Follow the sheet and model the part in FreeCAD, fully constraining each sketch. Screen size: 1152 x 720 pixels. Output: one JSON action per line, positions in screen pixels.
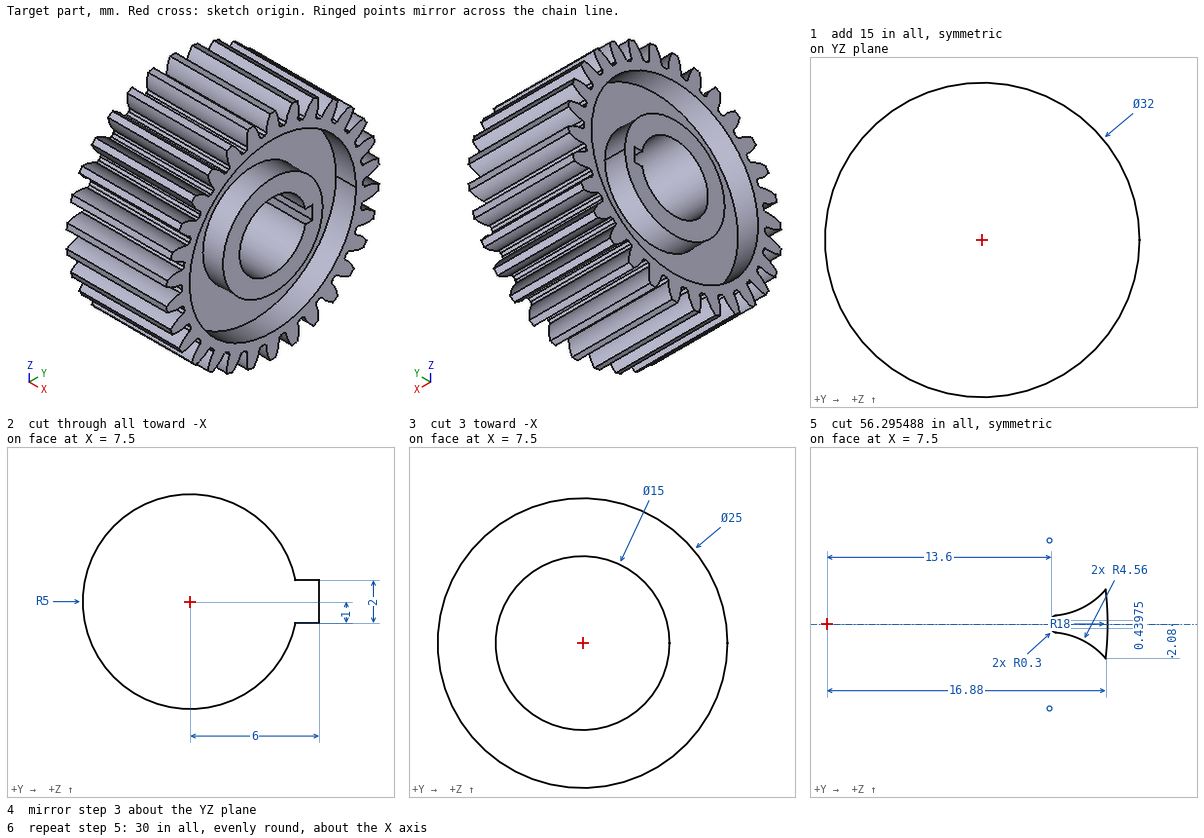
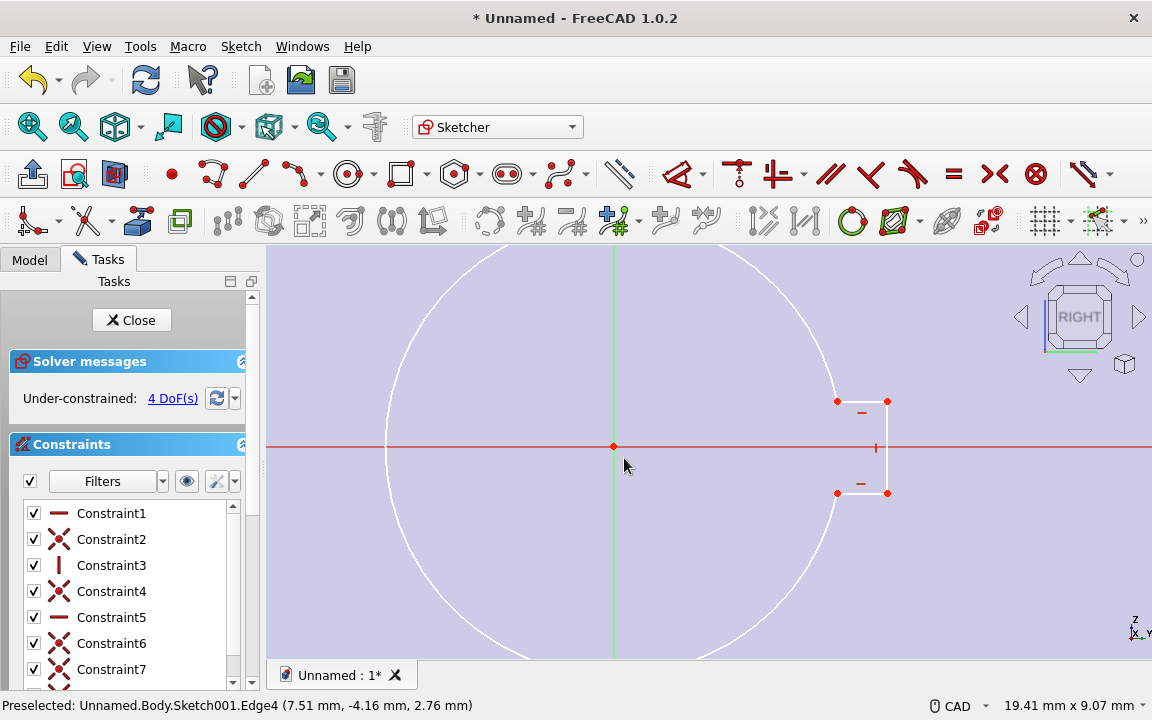
{"action": "left_click", "coordinate": [385, 446]}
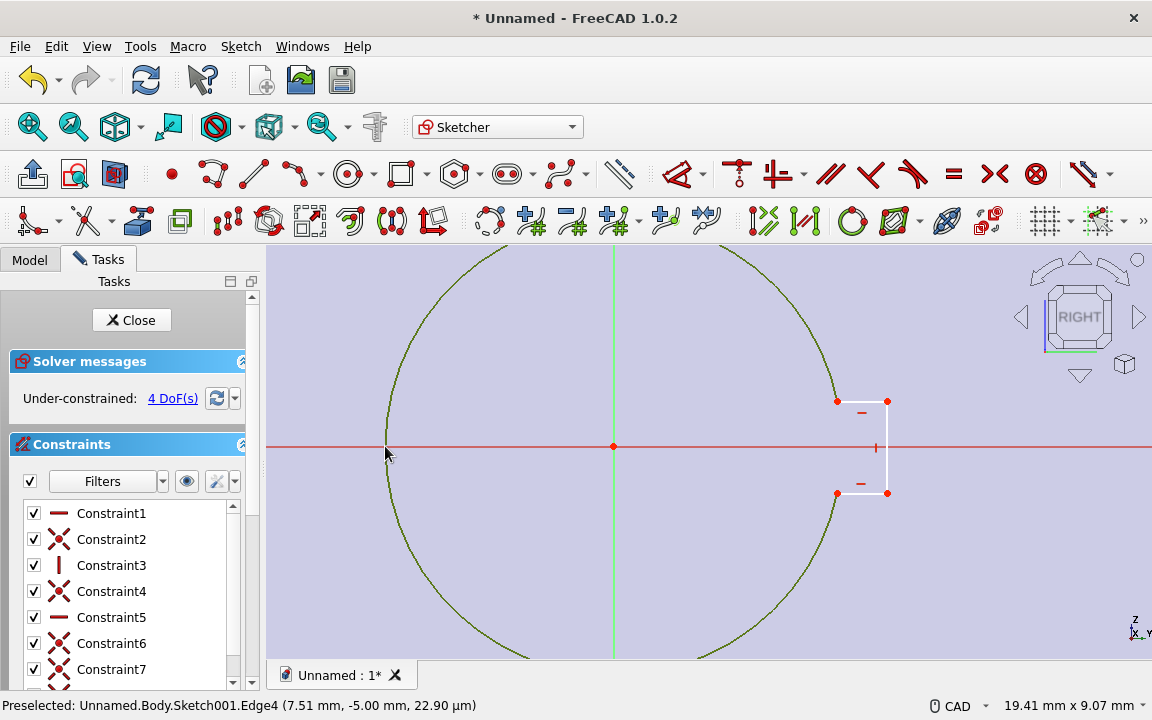
{"action": "key", "text": "k r"}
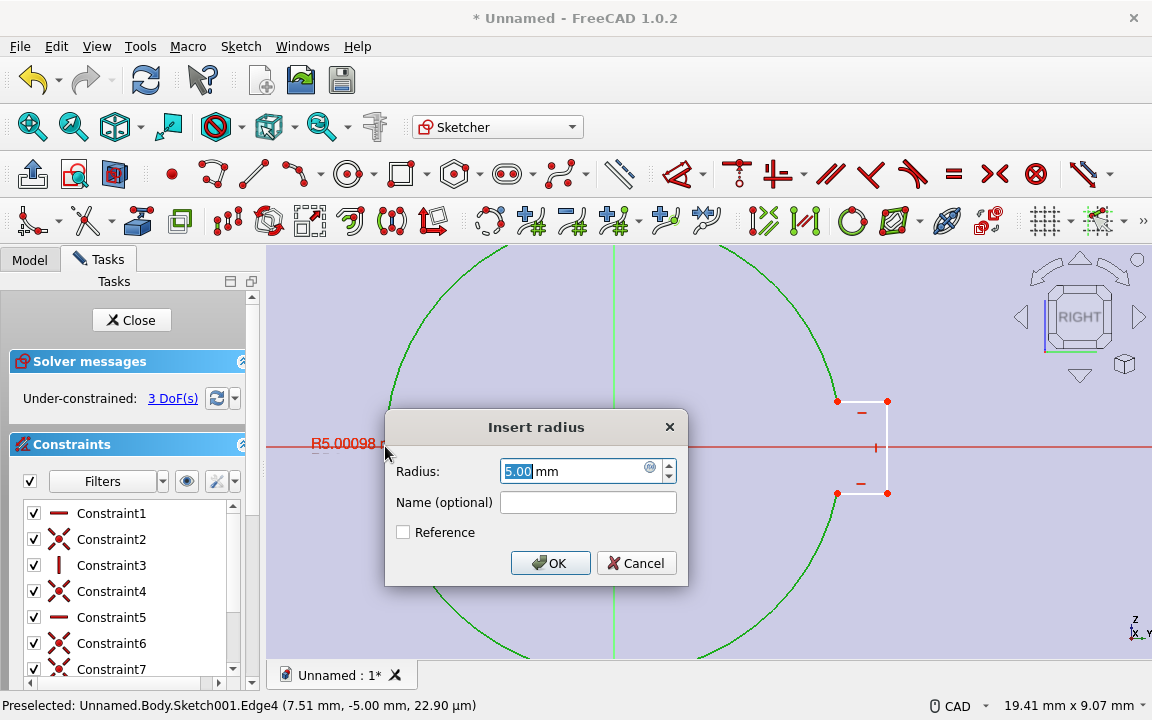
{"action": "type", "text": "5"}
{"action": "key", "text": "Return"}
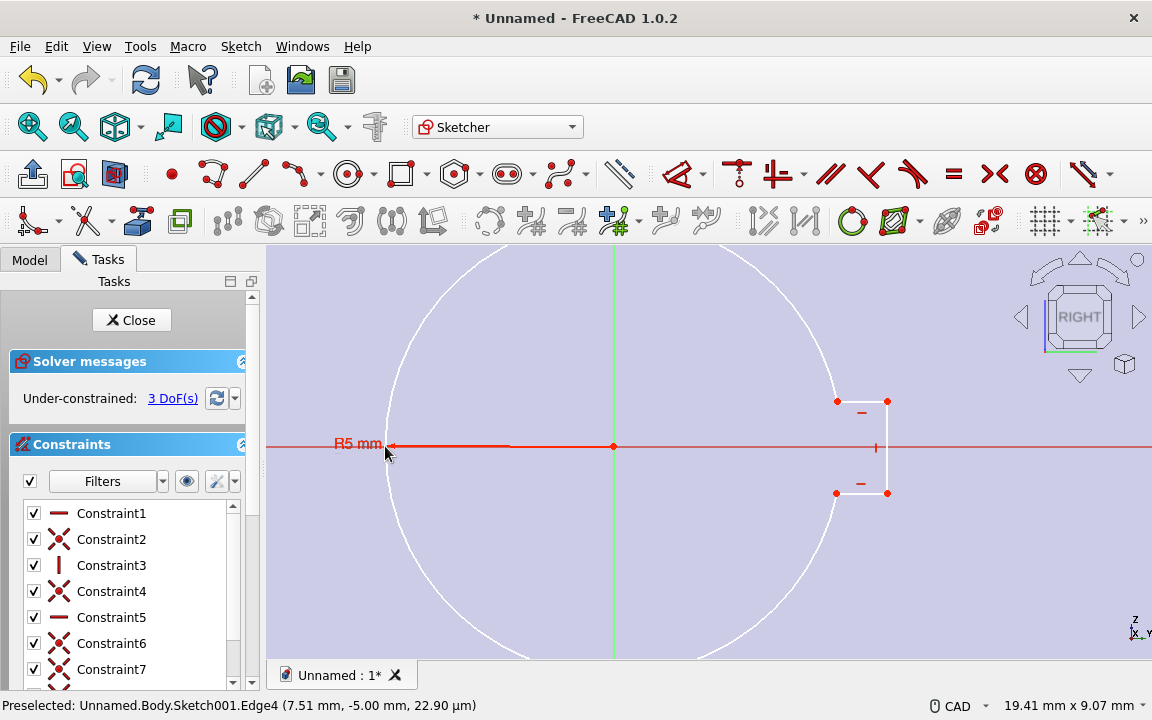
{"action": "left_click", "coordinate": [887, 466]}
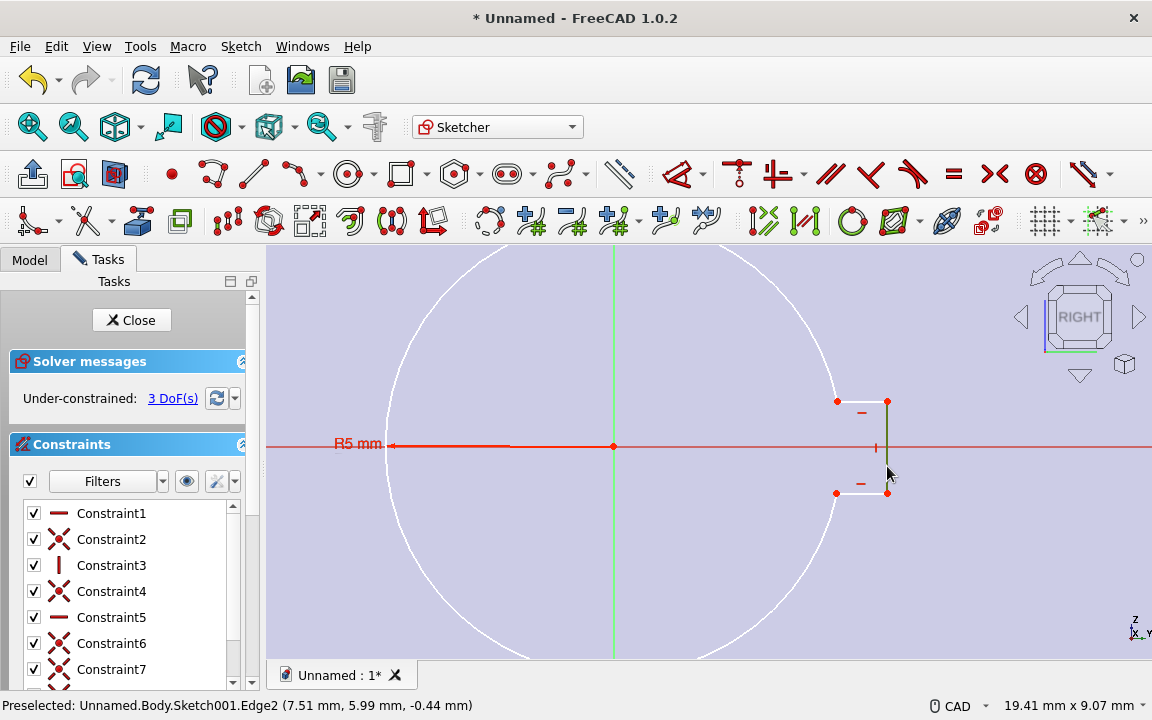
{"action": "key", "text": "i"}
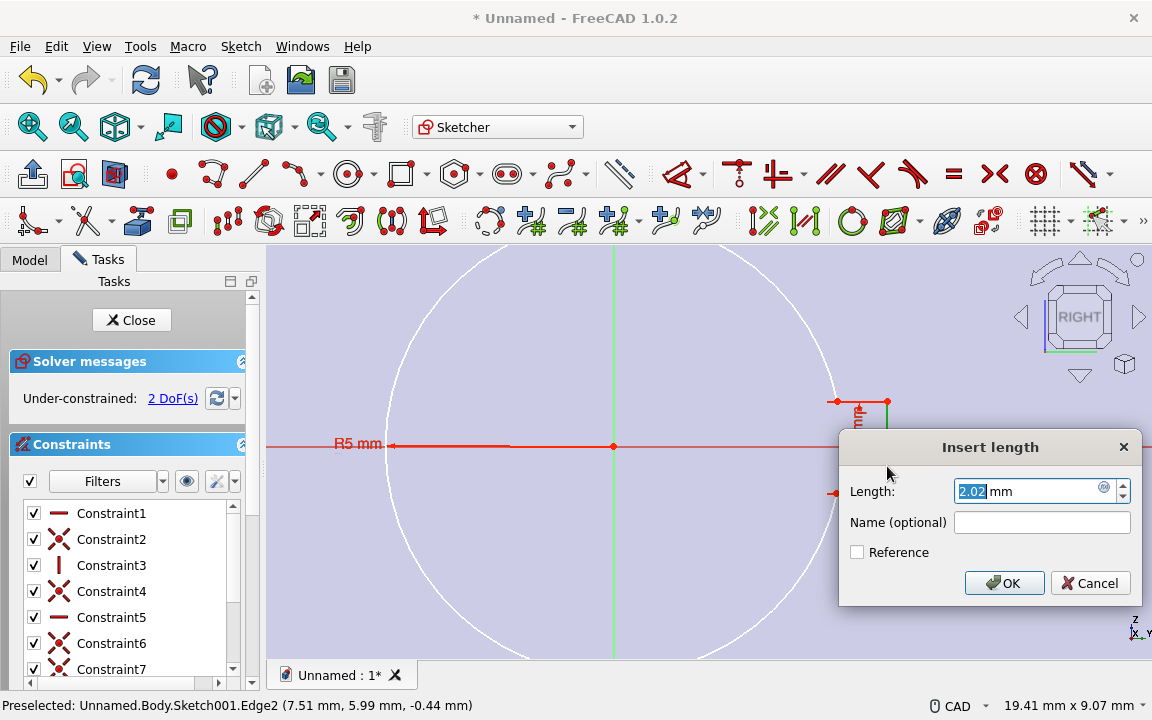
{"action": "type", "text": "2"}
{"action": "key", "text": "Return"}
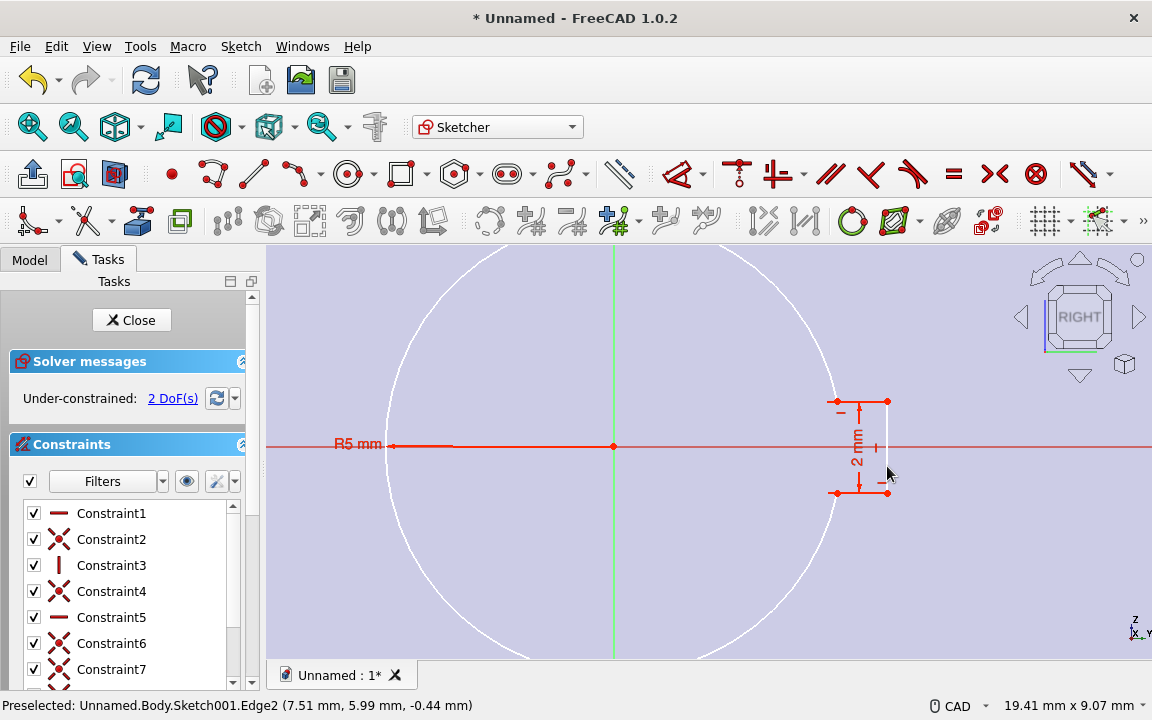
{"action": "left_click", "coordinate": [837, 493]}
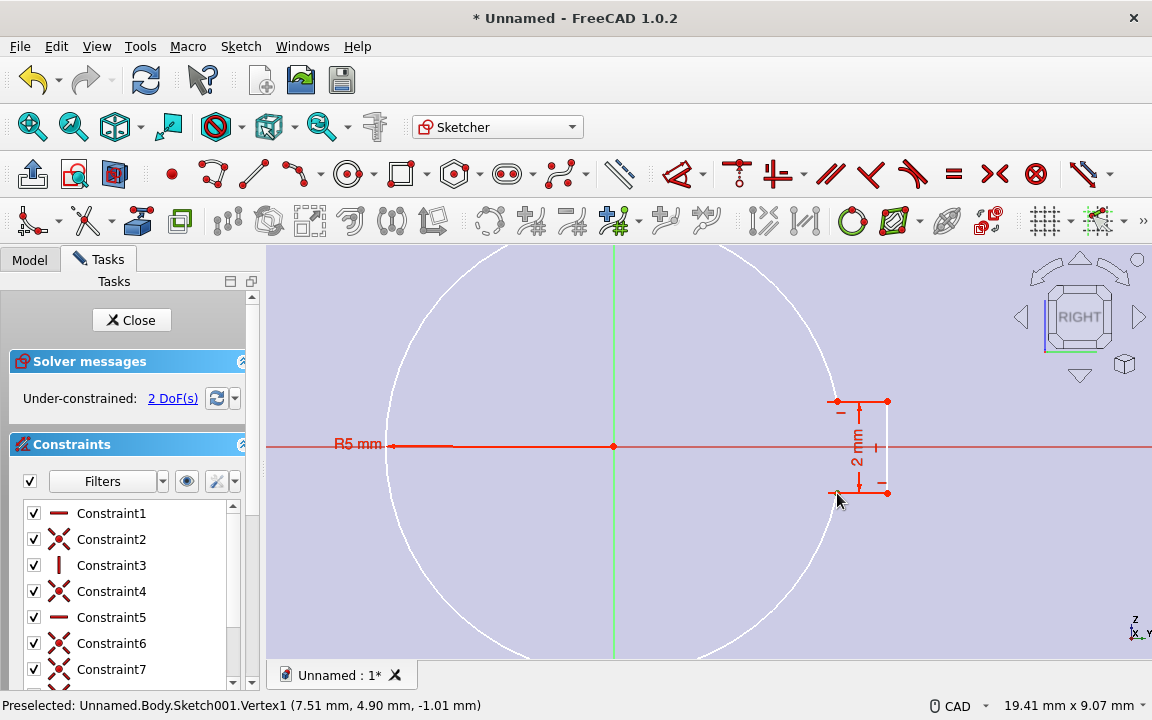
{"action": "key", "text": "i"}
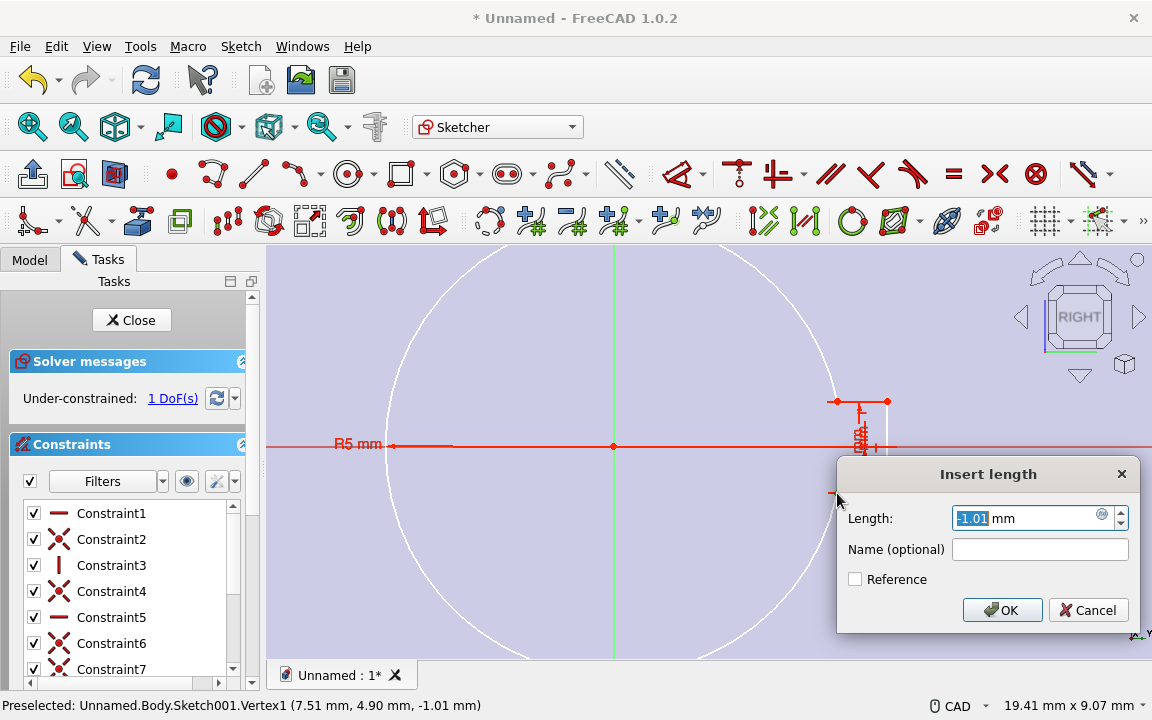
{"action": "type", "text": "-1"}
{"action": "key", "text": "Return"}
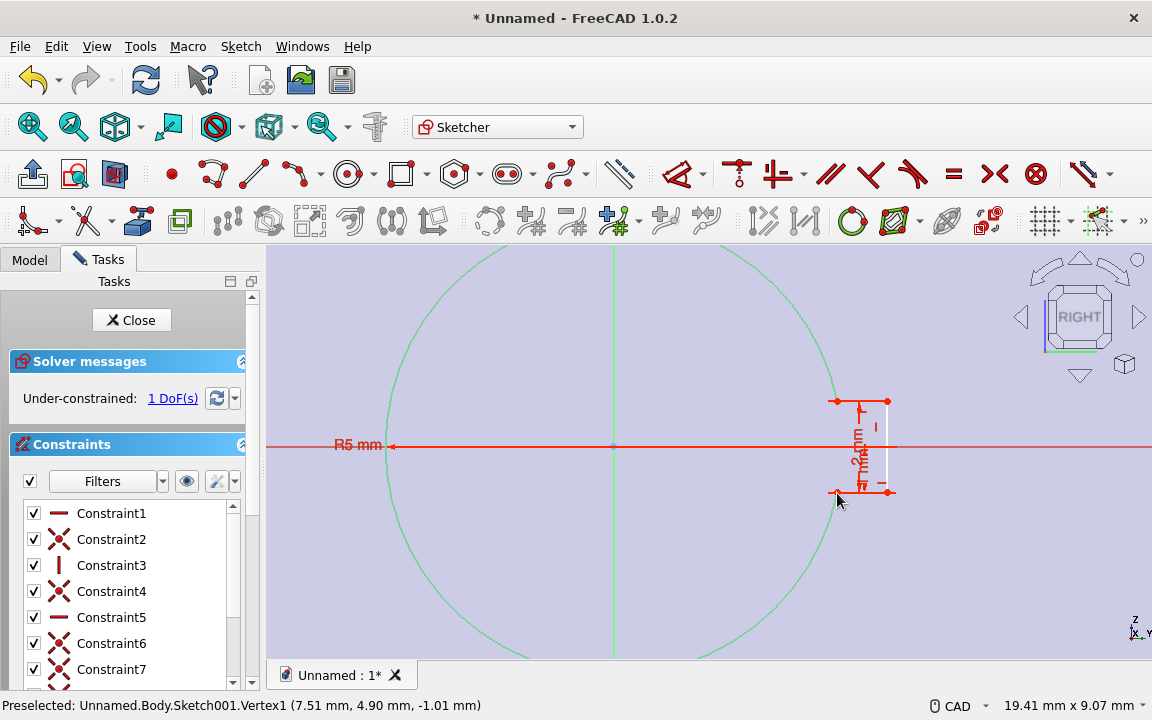
{"action": "left_click", "coordinate": [887, 493]}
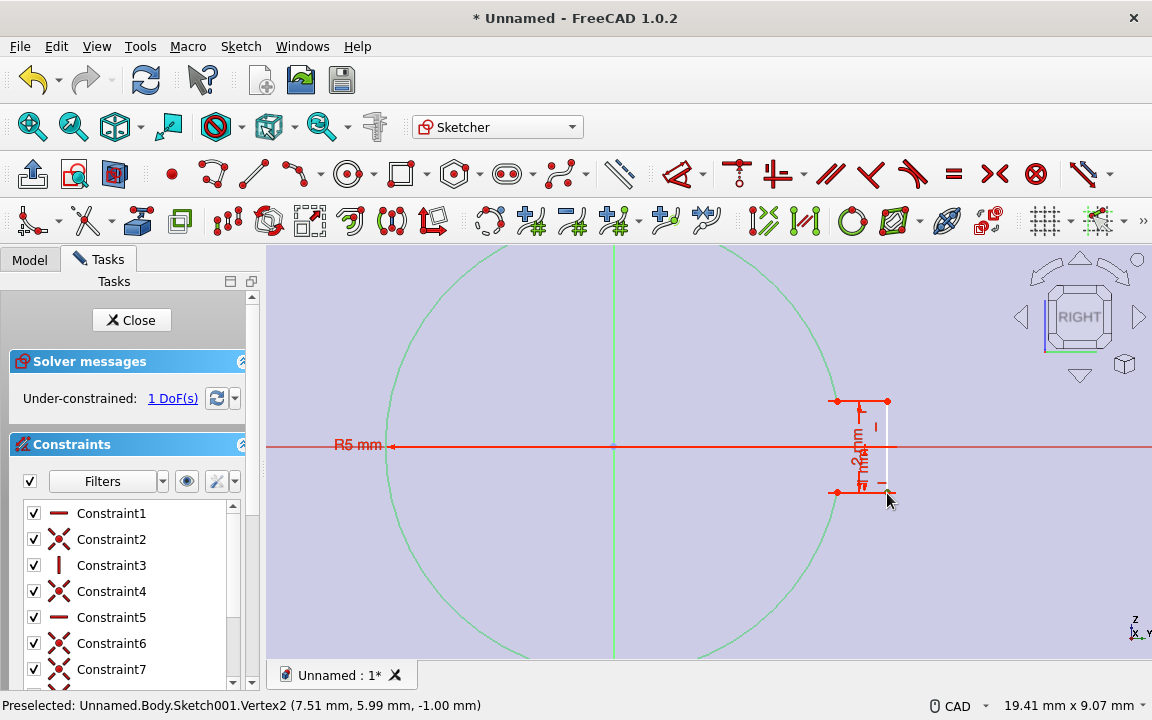
{"action": "key", "text": "l"}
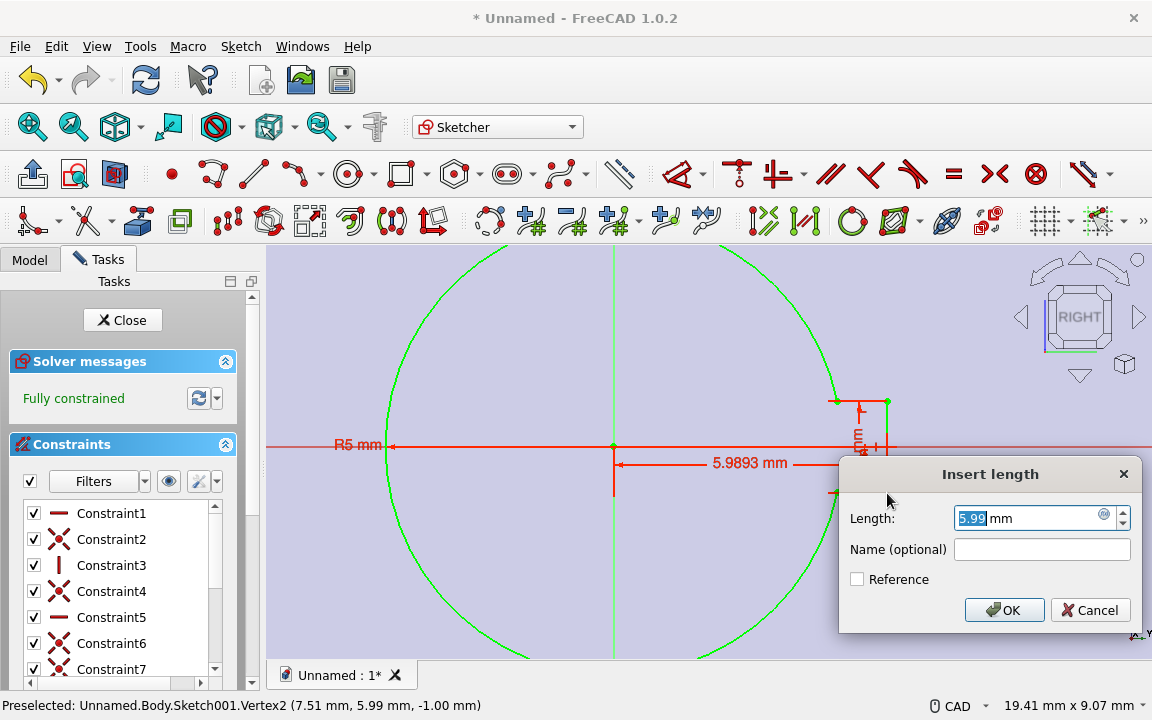
{"action": "type", "text": "6"}
{"action": "key", "text": "Return"}